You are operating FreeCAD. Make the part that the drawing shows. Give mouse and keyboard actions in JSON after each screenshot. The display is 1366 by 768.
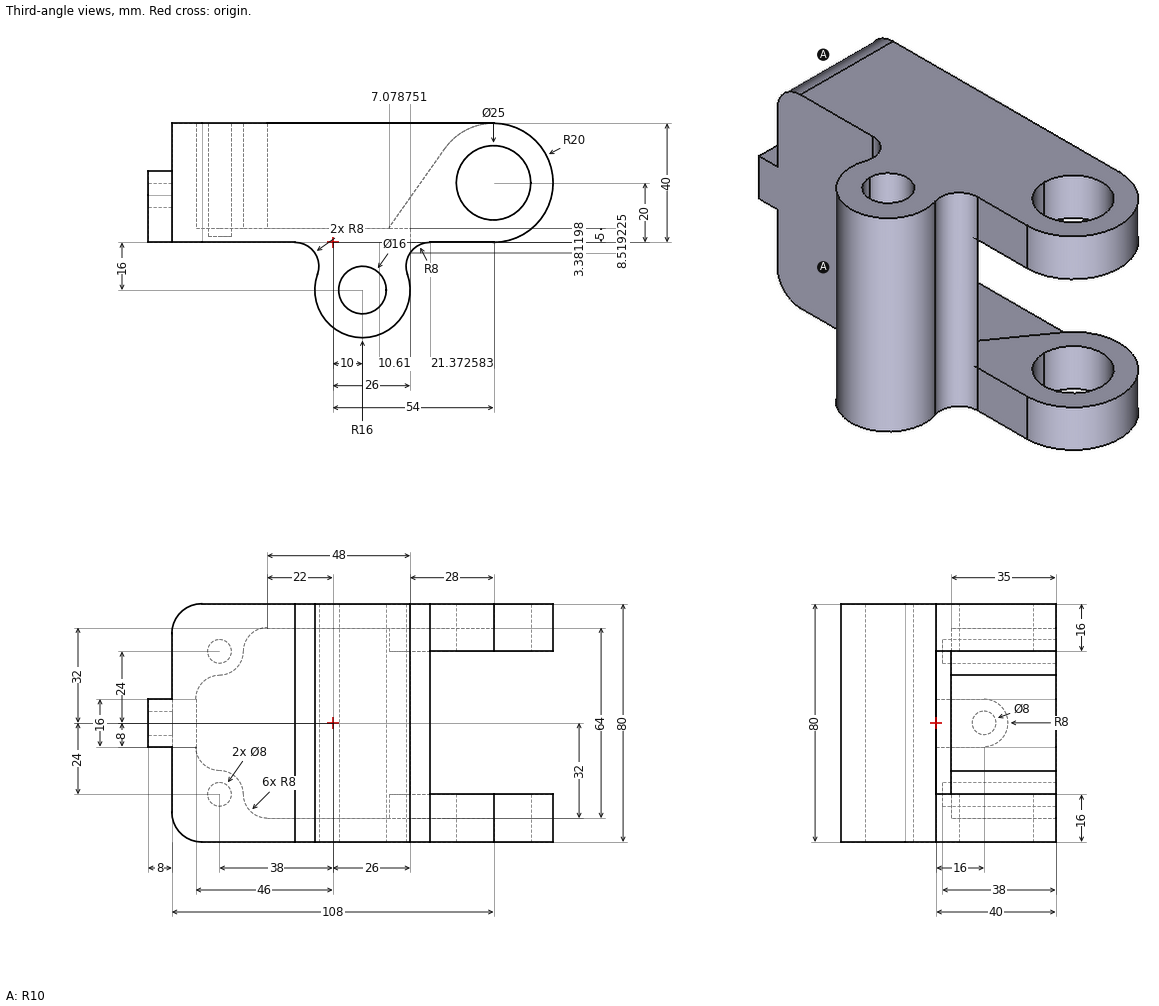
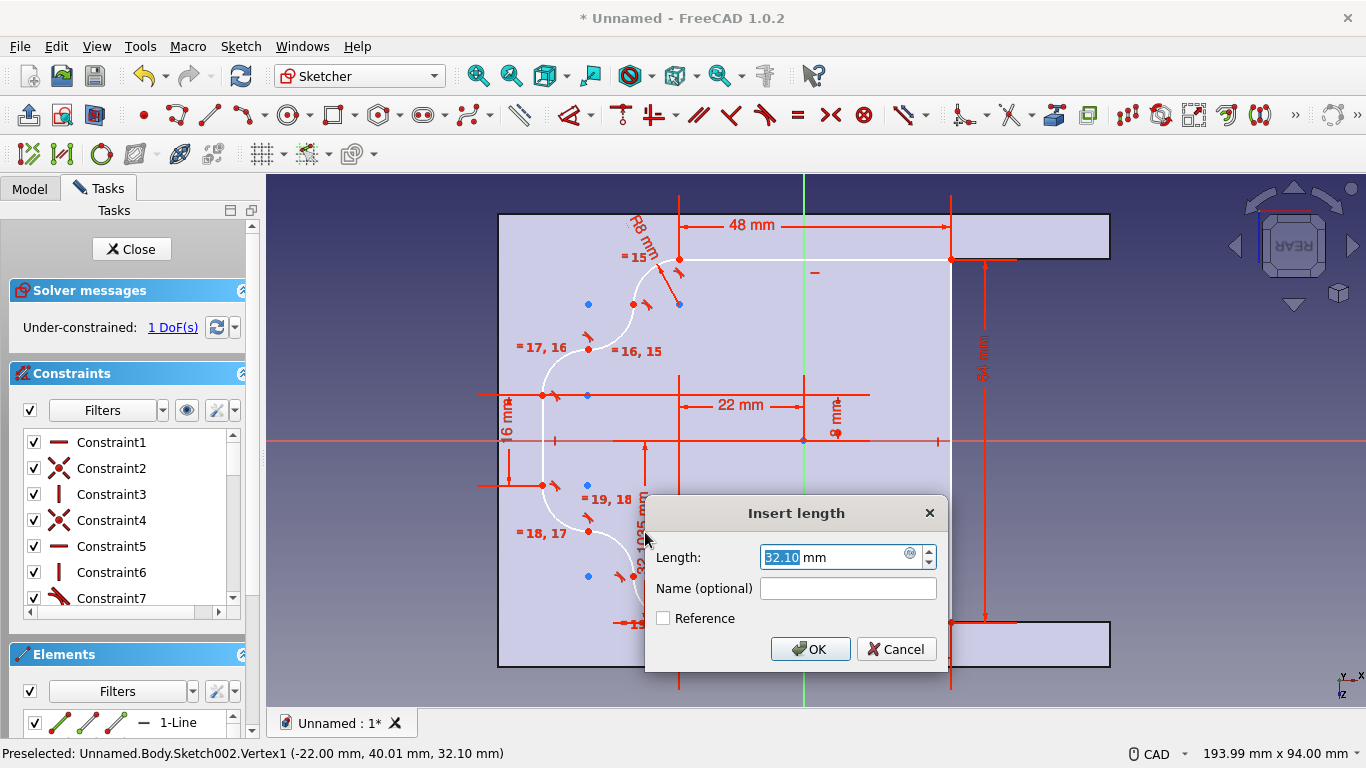
{"action": "type", "text": "32"}
{"action": "key", "text": "Return"}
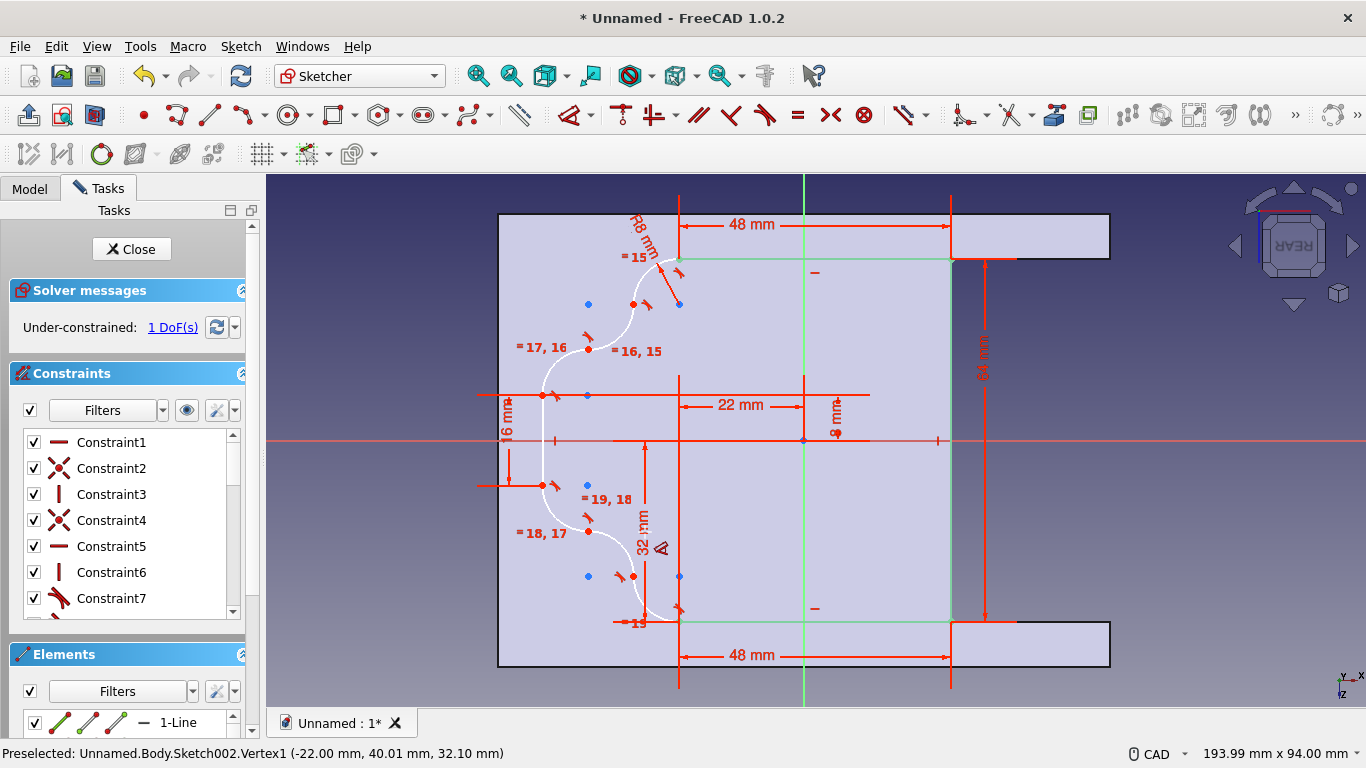
{"action": "left_click", "coordinate": [543, 395]}
{"action": "left_click", "coordinate": [673, 361]}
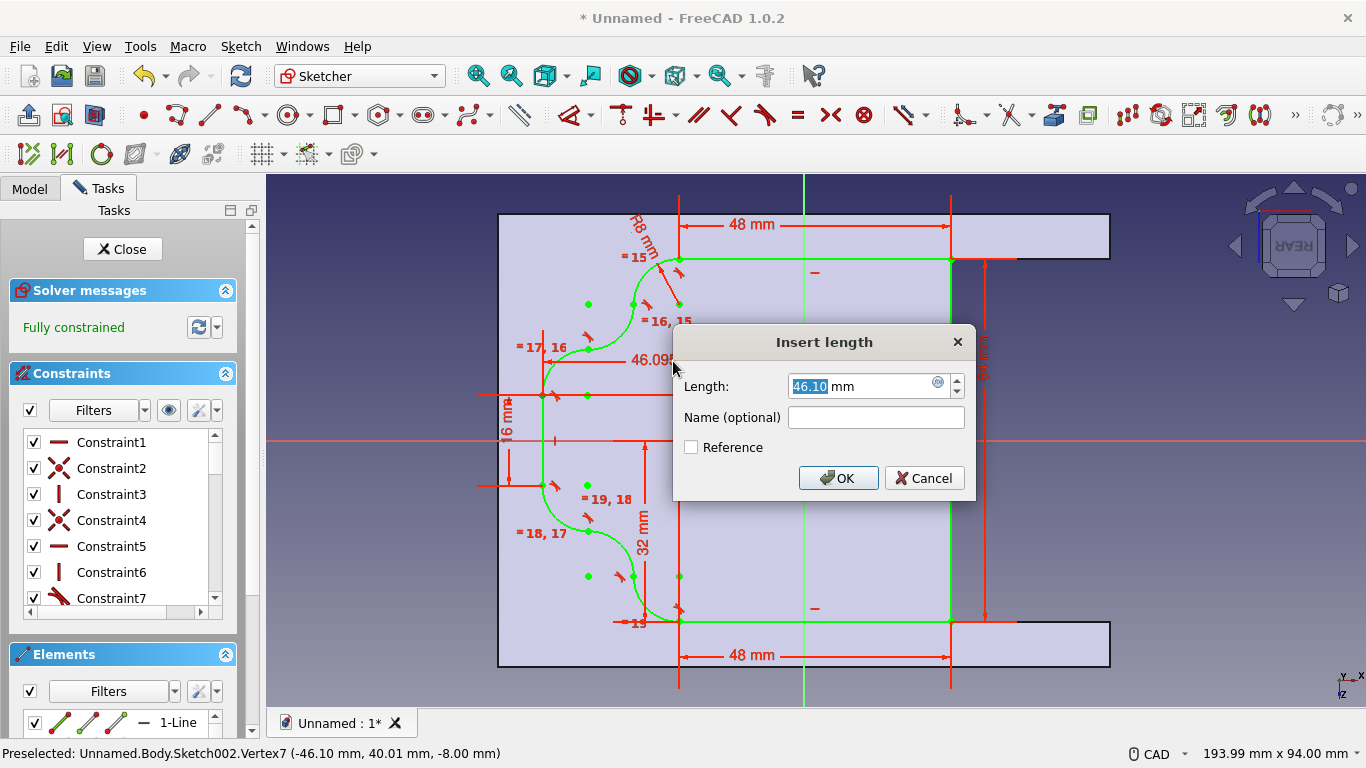
{"action": "type", "text": "46"}
{"action": "key", "text": "Return"}
{"action": "key", "text": "Escape"}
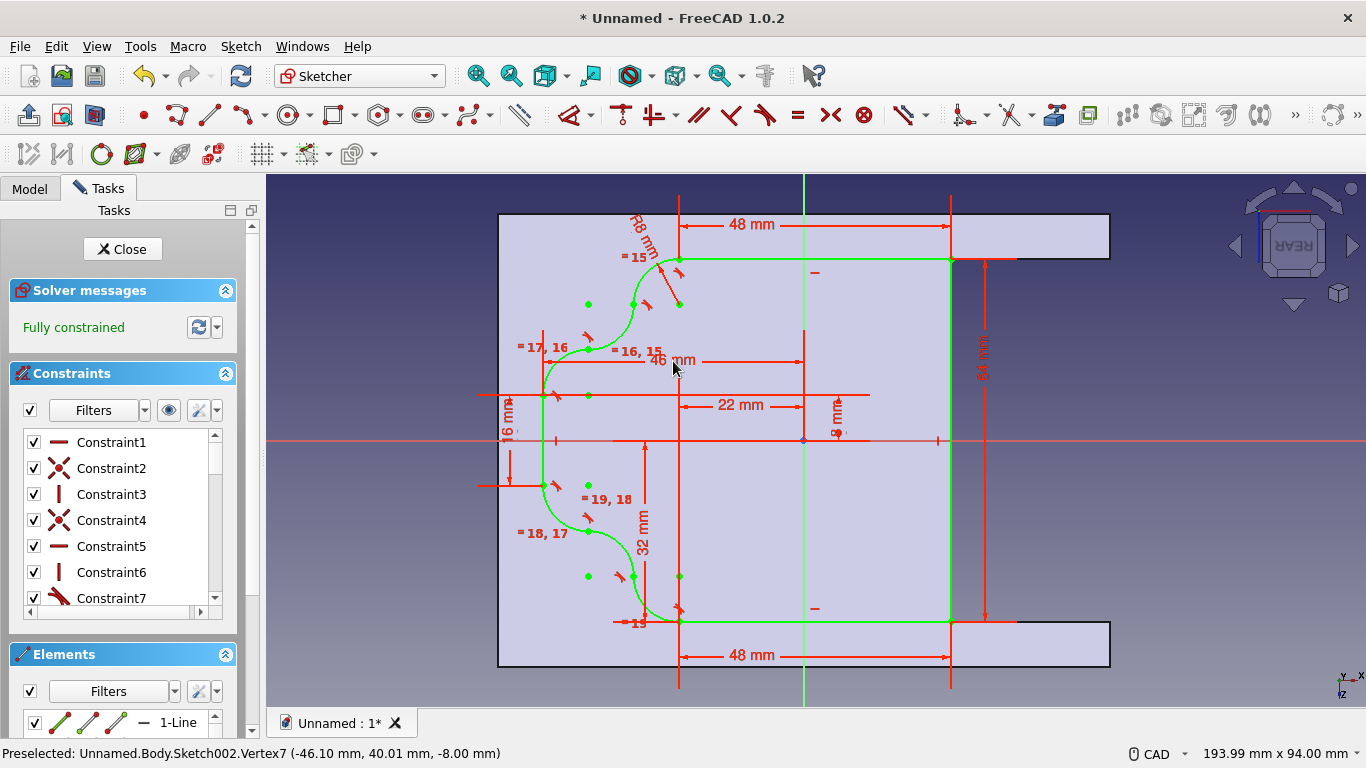
{"action": "left_click", "coordinate": [123, 249]}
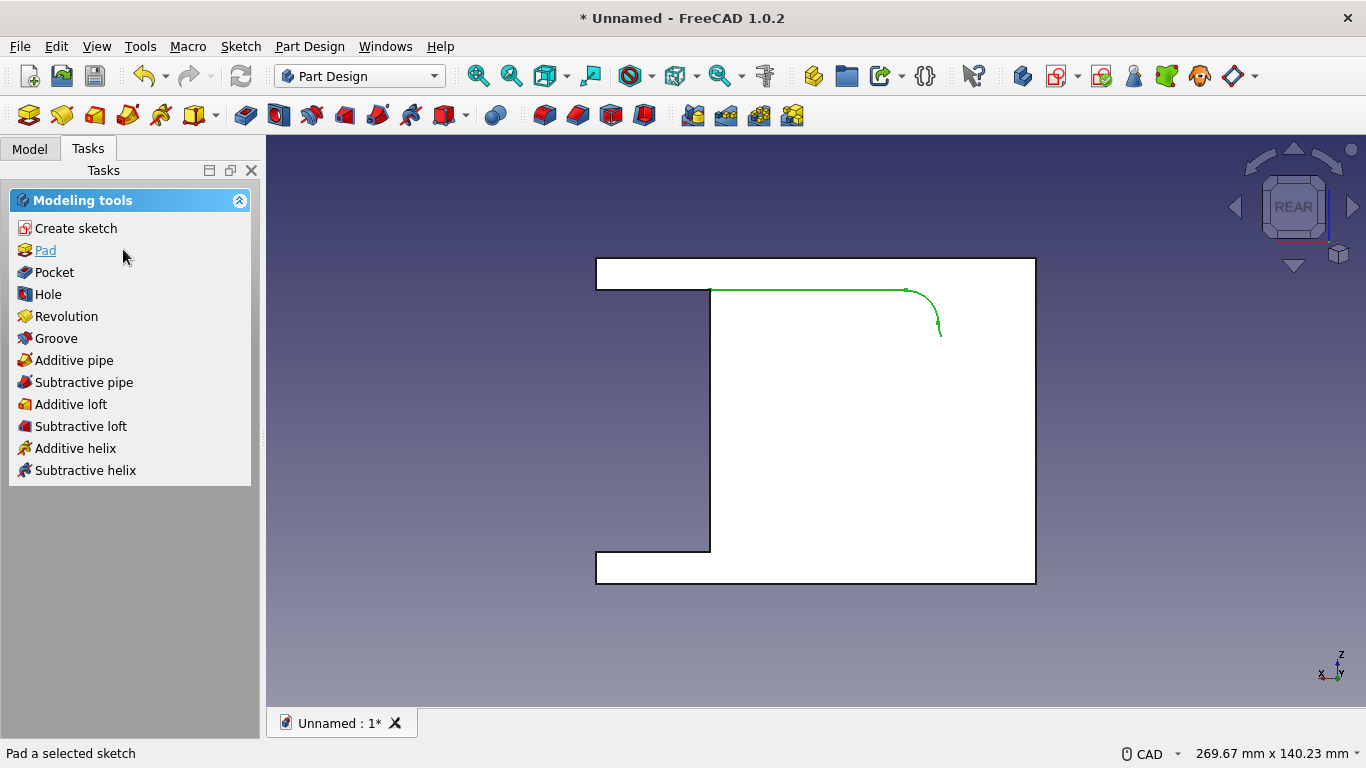
{"action": "left_click", "coordinate": [246, 116]}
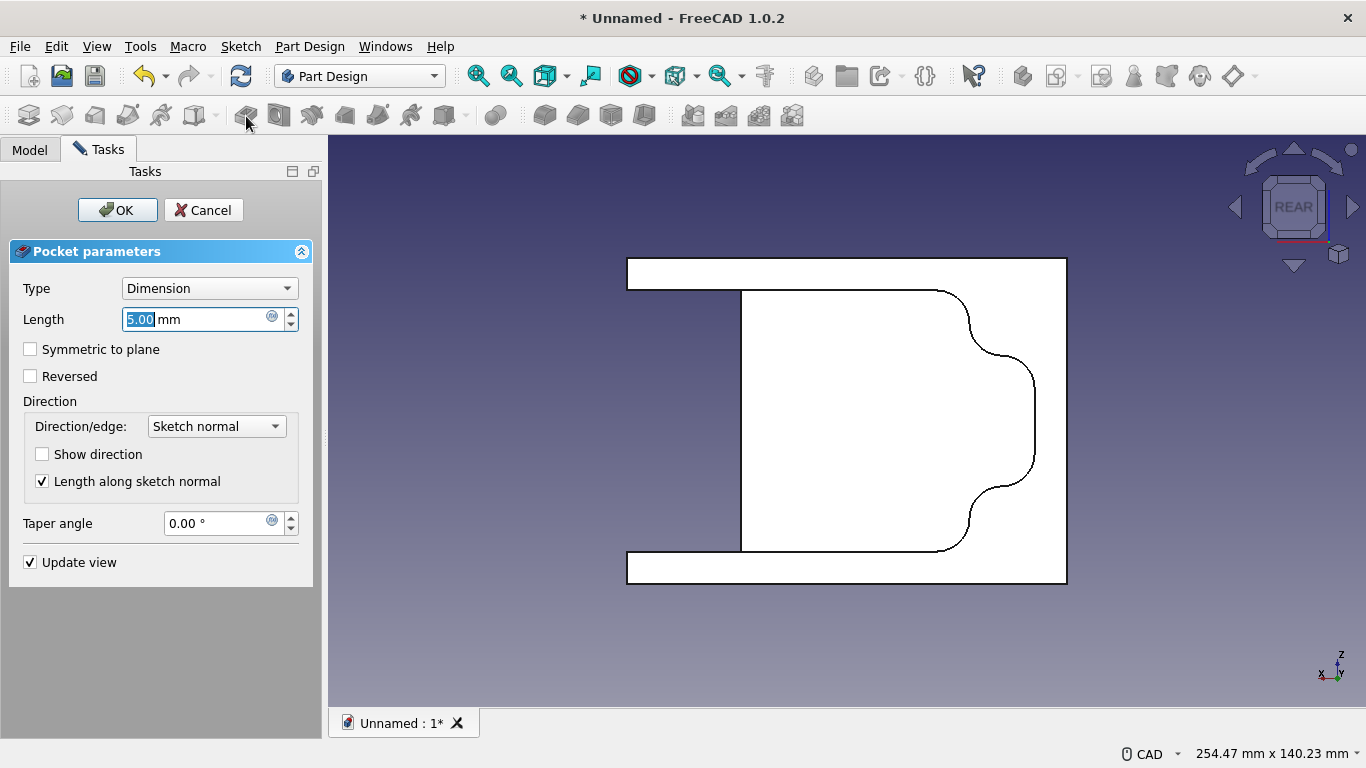
{"action": "type", "text": "35"}
{"action": "key", "text": "Tab"}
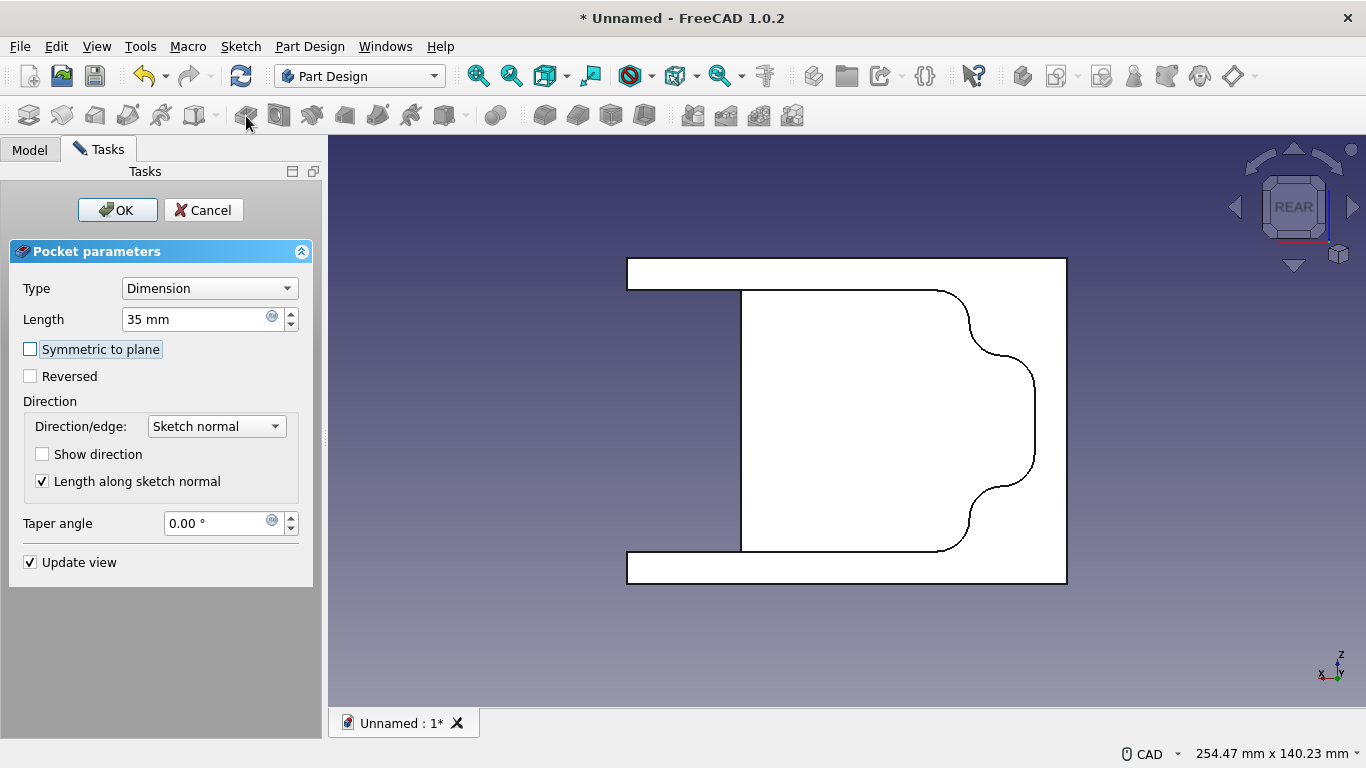
{"action": "left_click", "coordinate": [118, 210]}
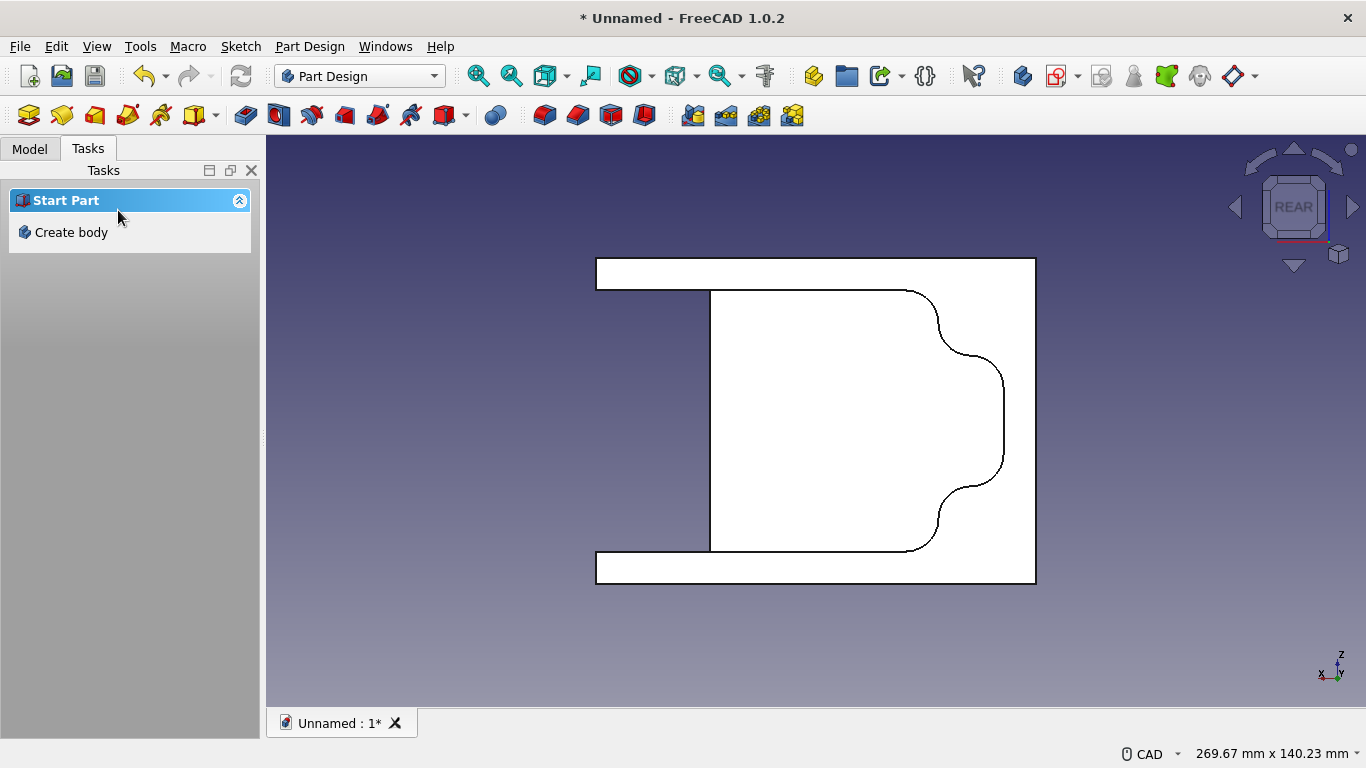
{"action": "key", "text": "0"}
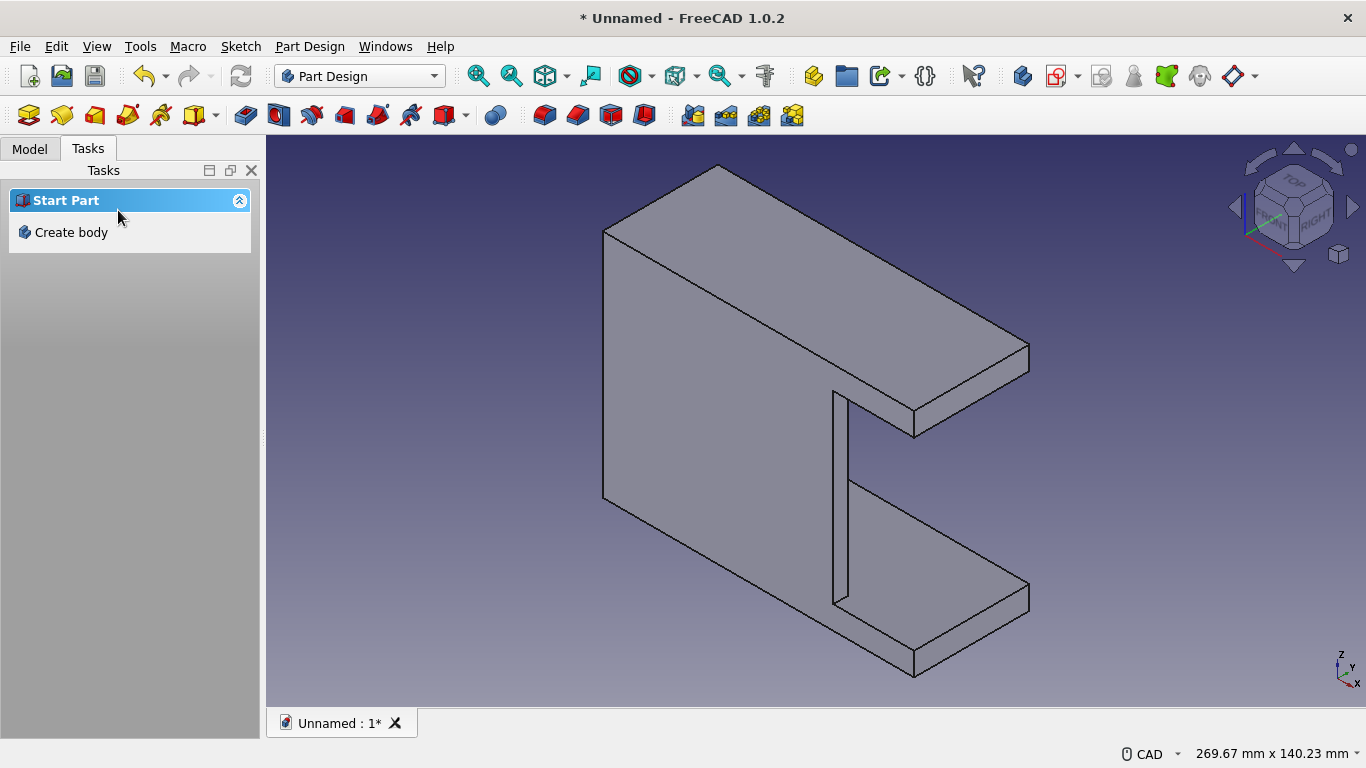
{"action": "left_click", "coordinate": [905, 338]}